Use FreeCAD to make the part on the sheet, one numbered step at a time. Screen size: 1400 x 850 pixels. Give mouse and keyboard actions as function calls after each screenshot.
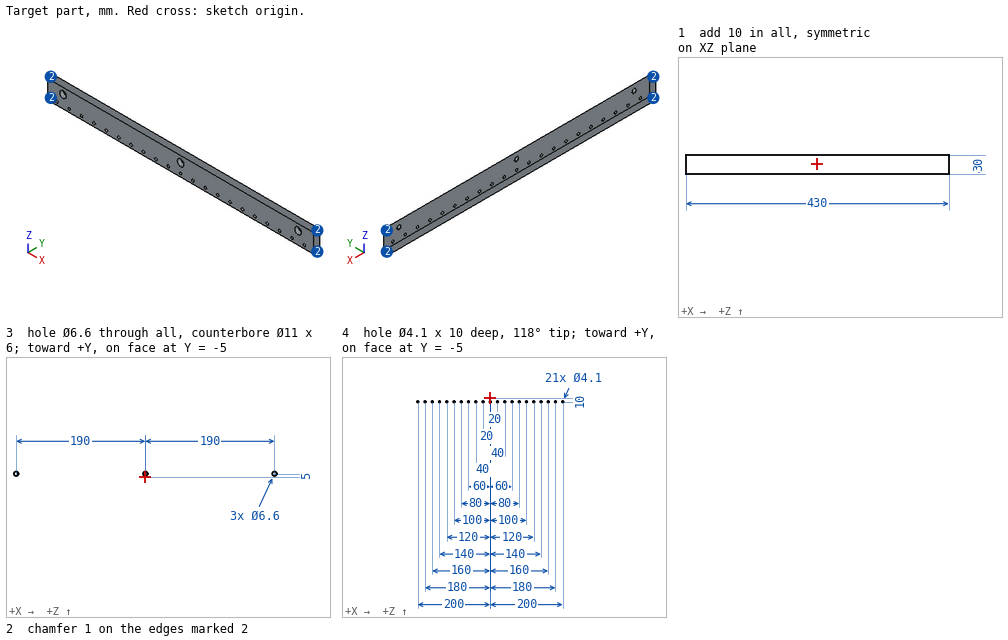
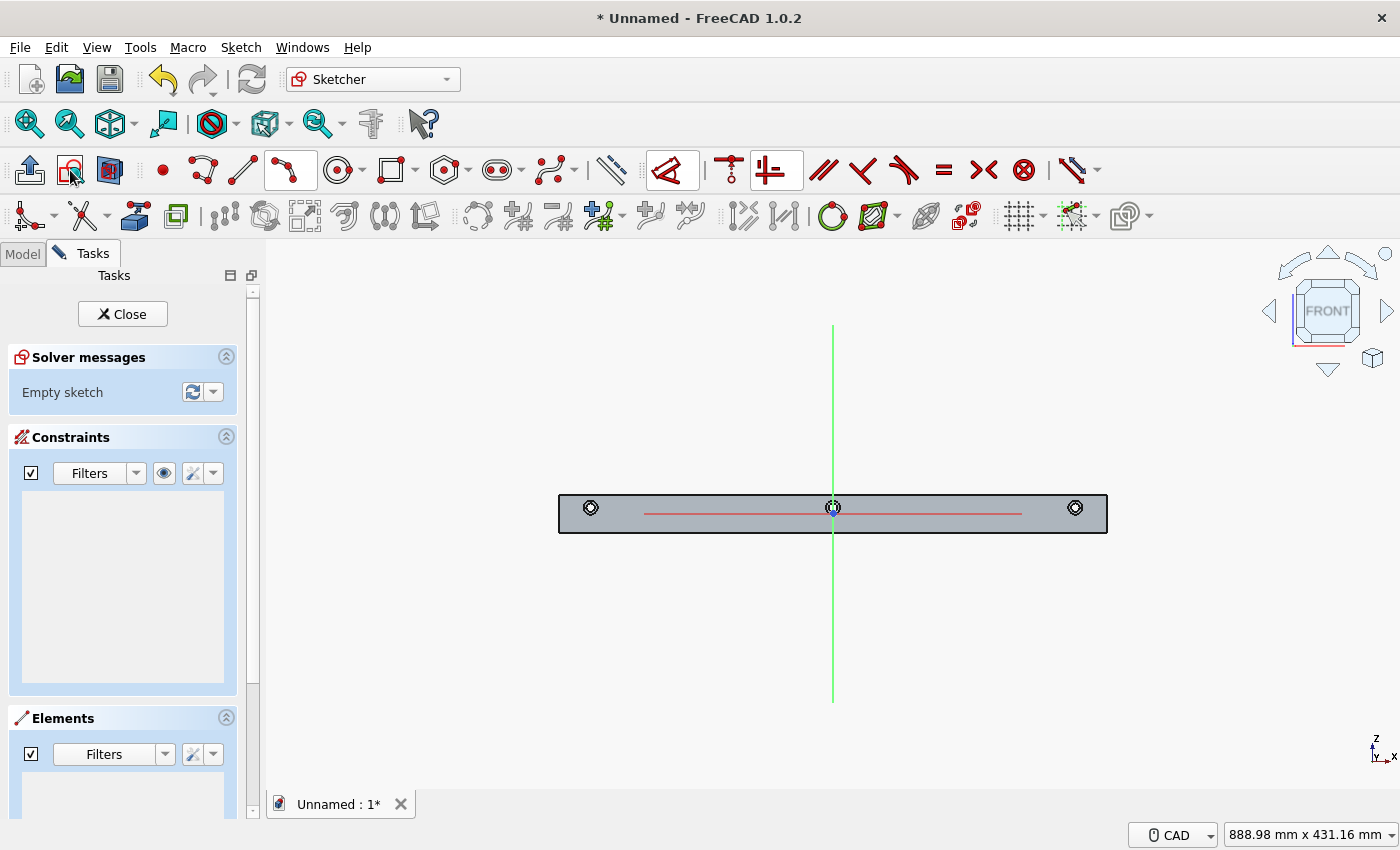
click(338, 170)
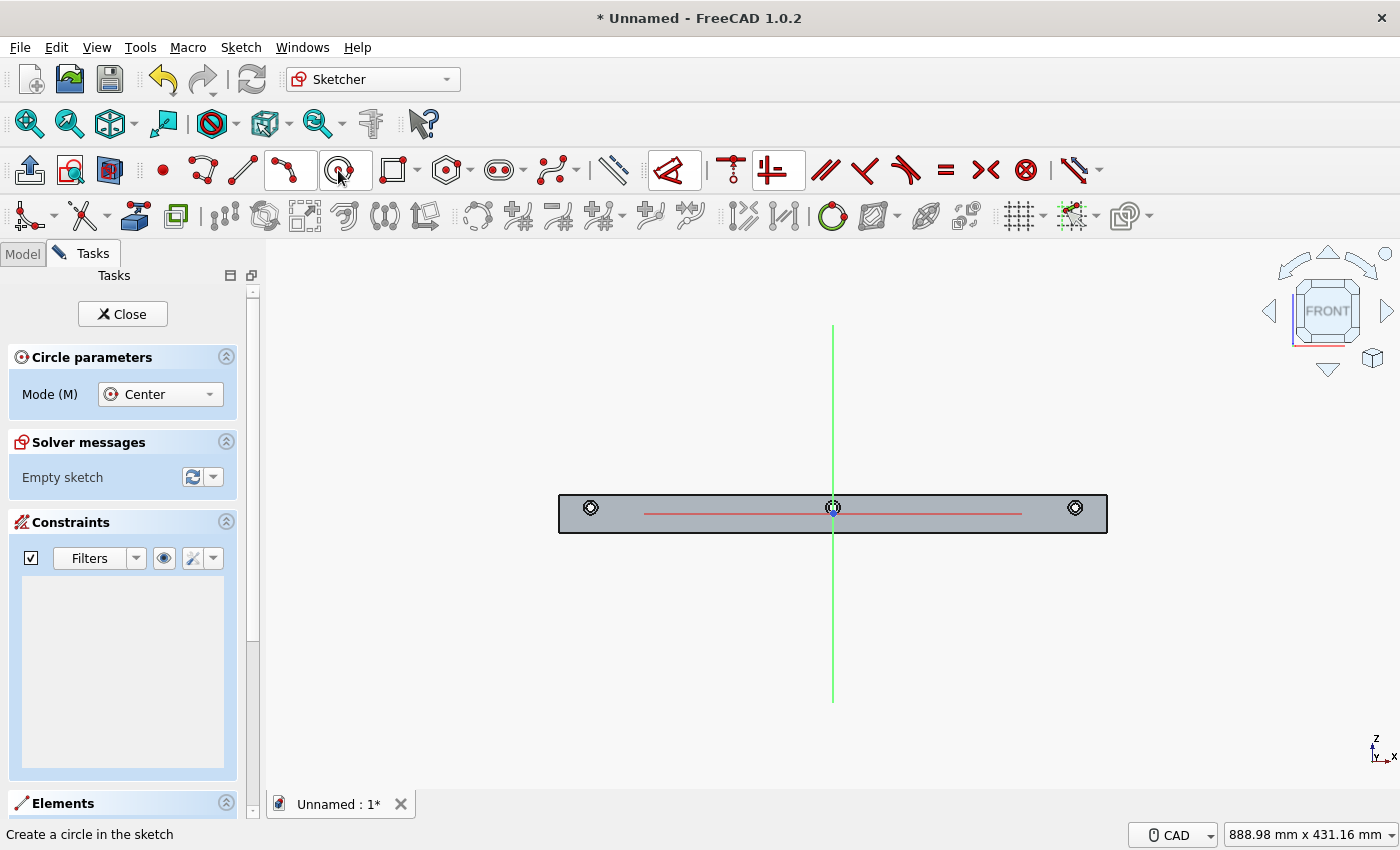
scroll(1088, 527, up, 11)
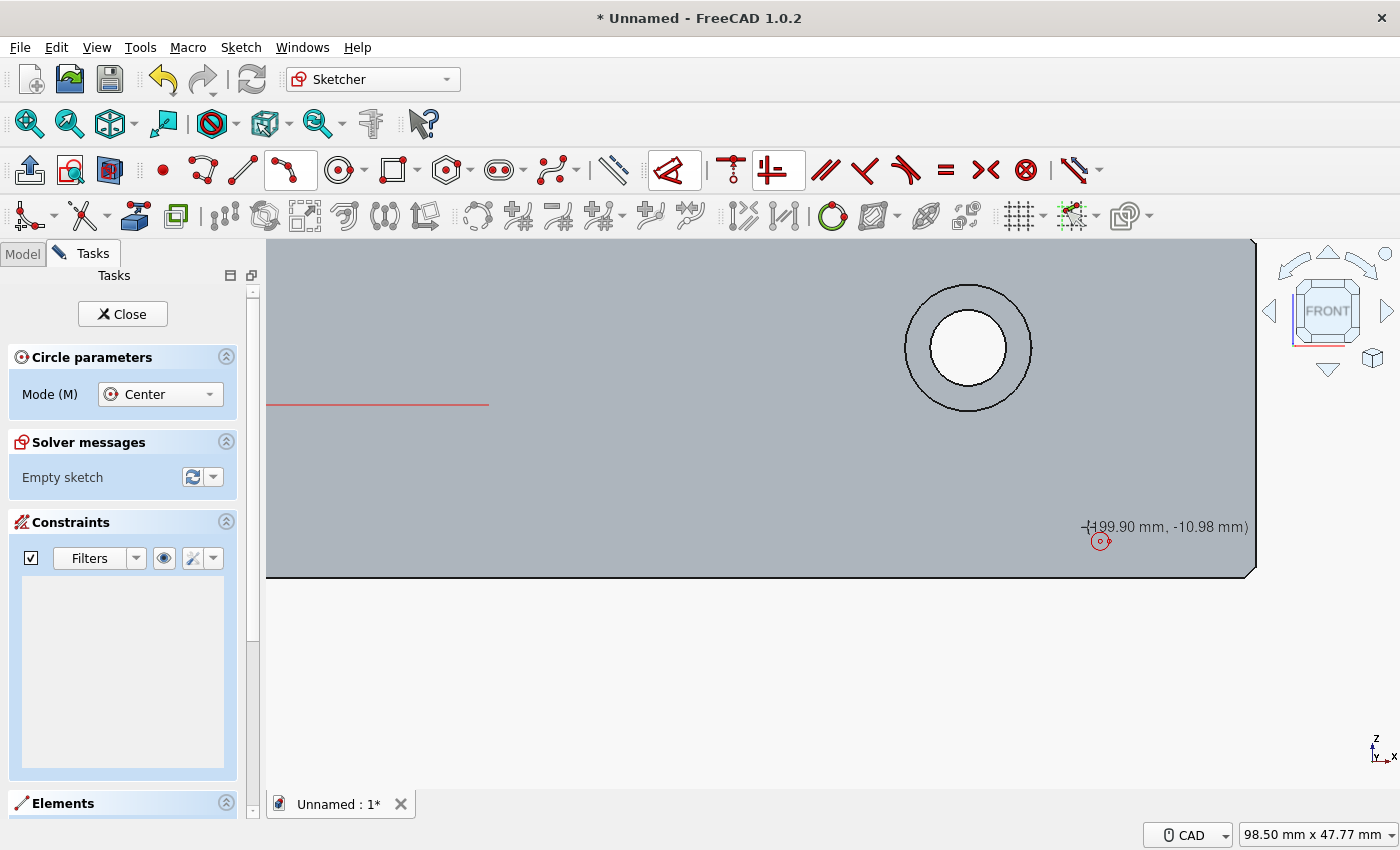
scroll(1075, 520, down, 10)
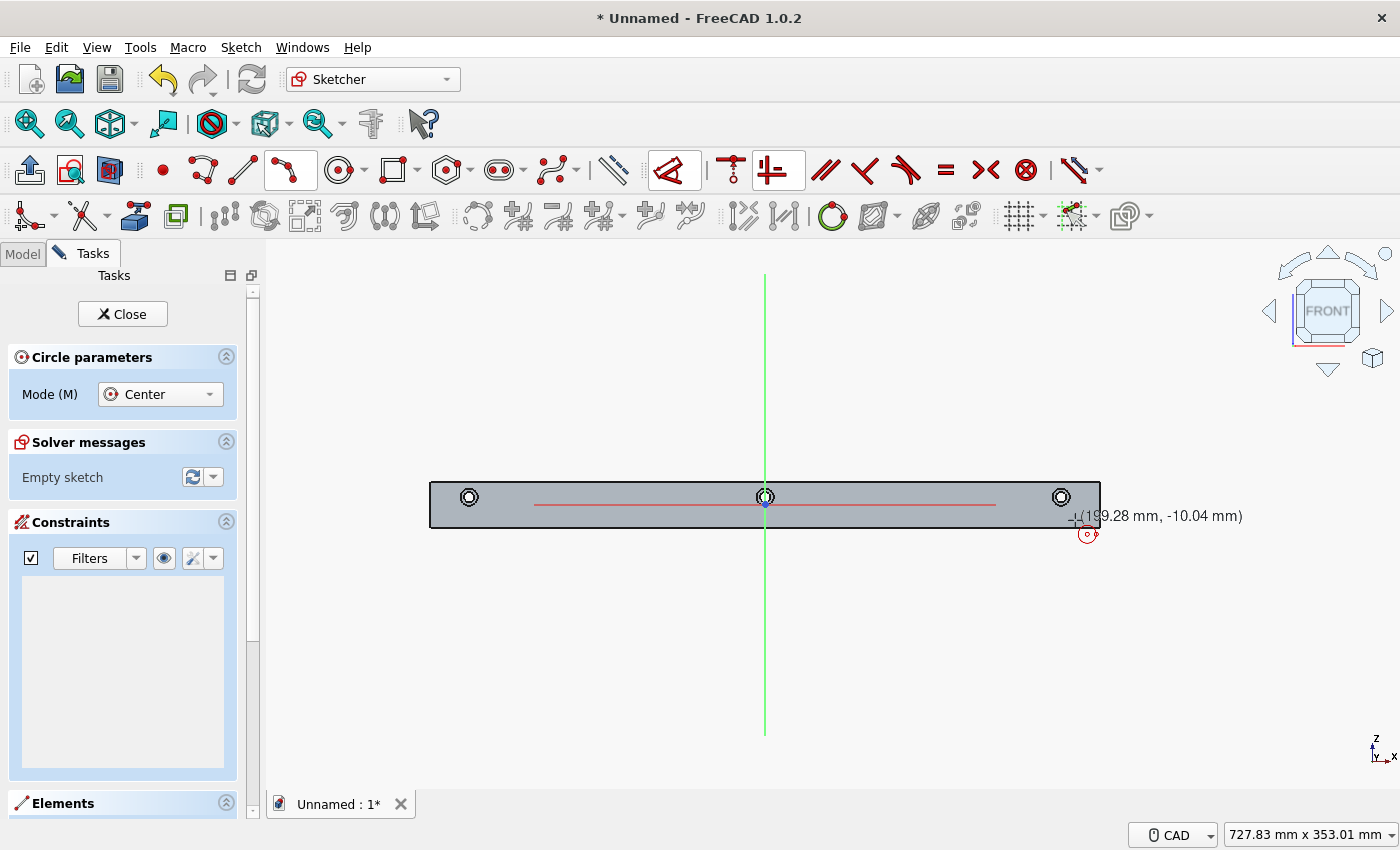
click(1077, 521)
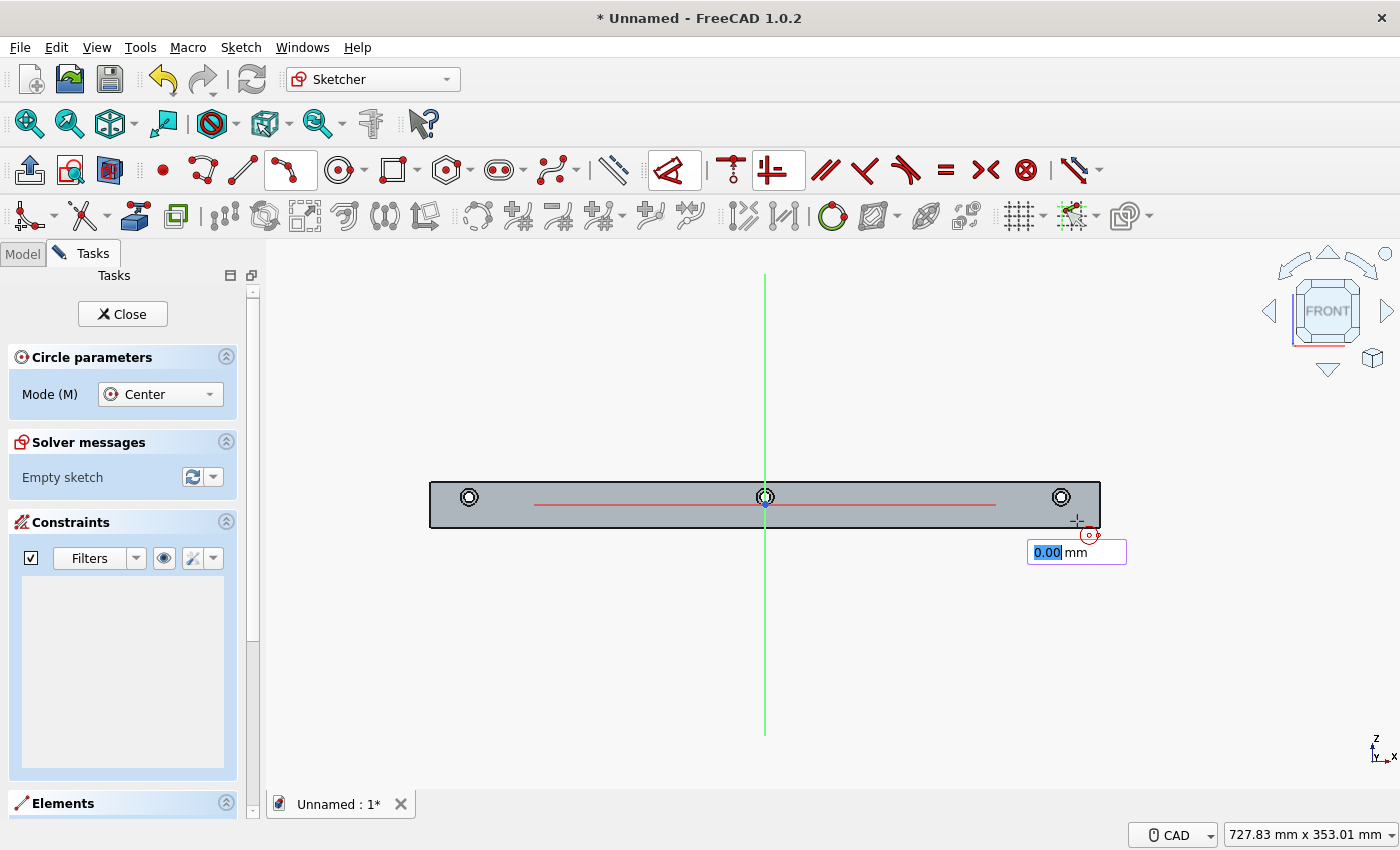
scroll(1079, 523, up, 9)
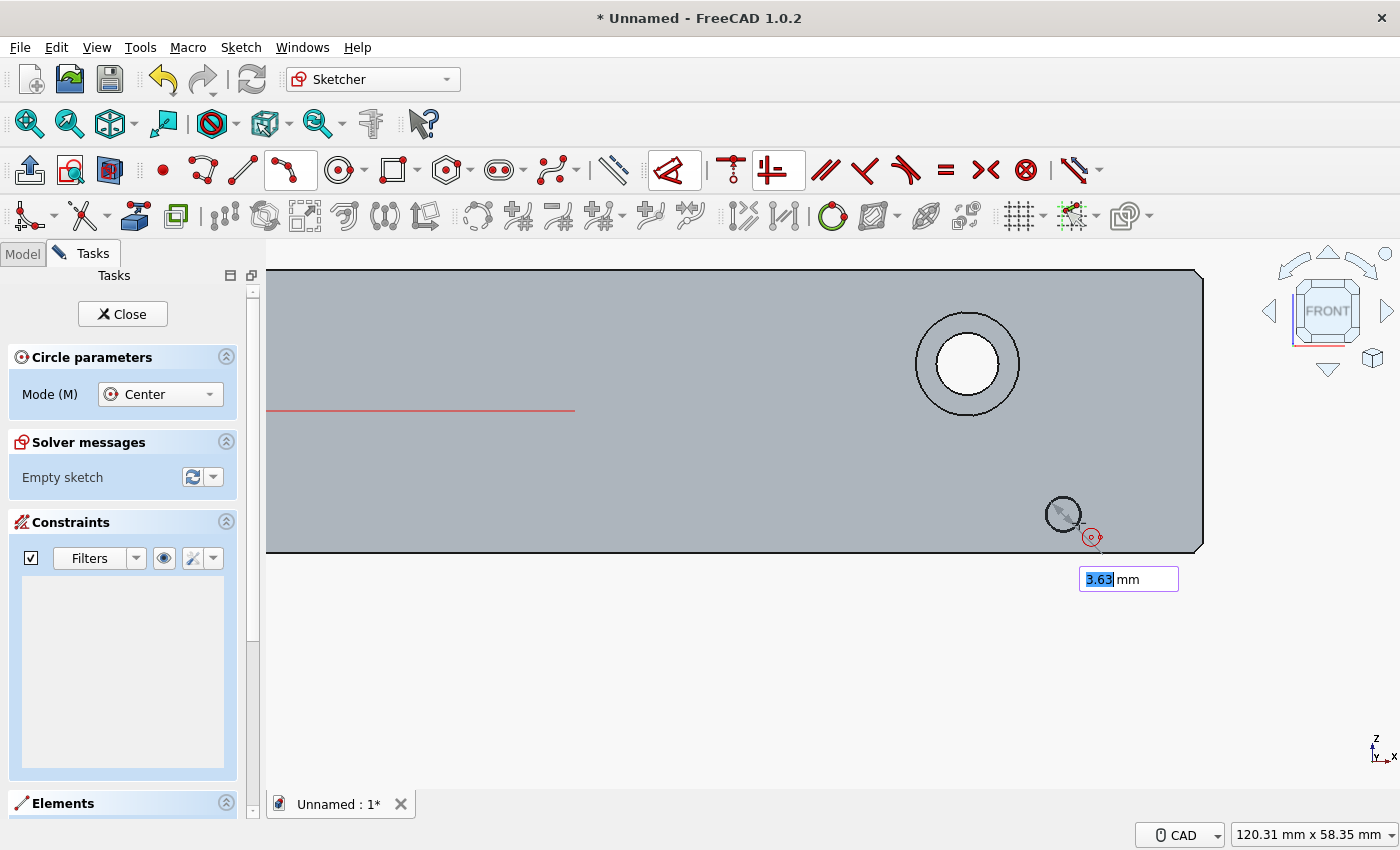
click(1075, 519)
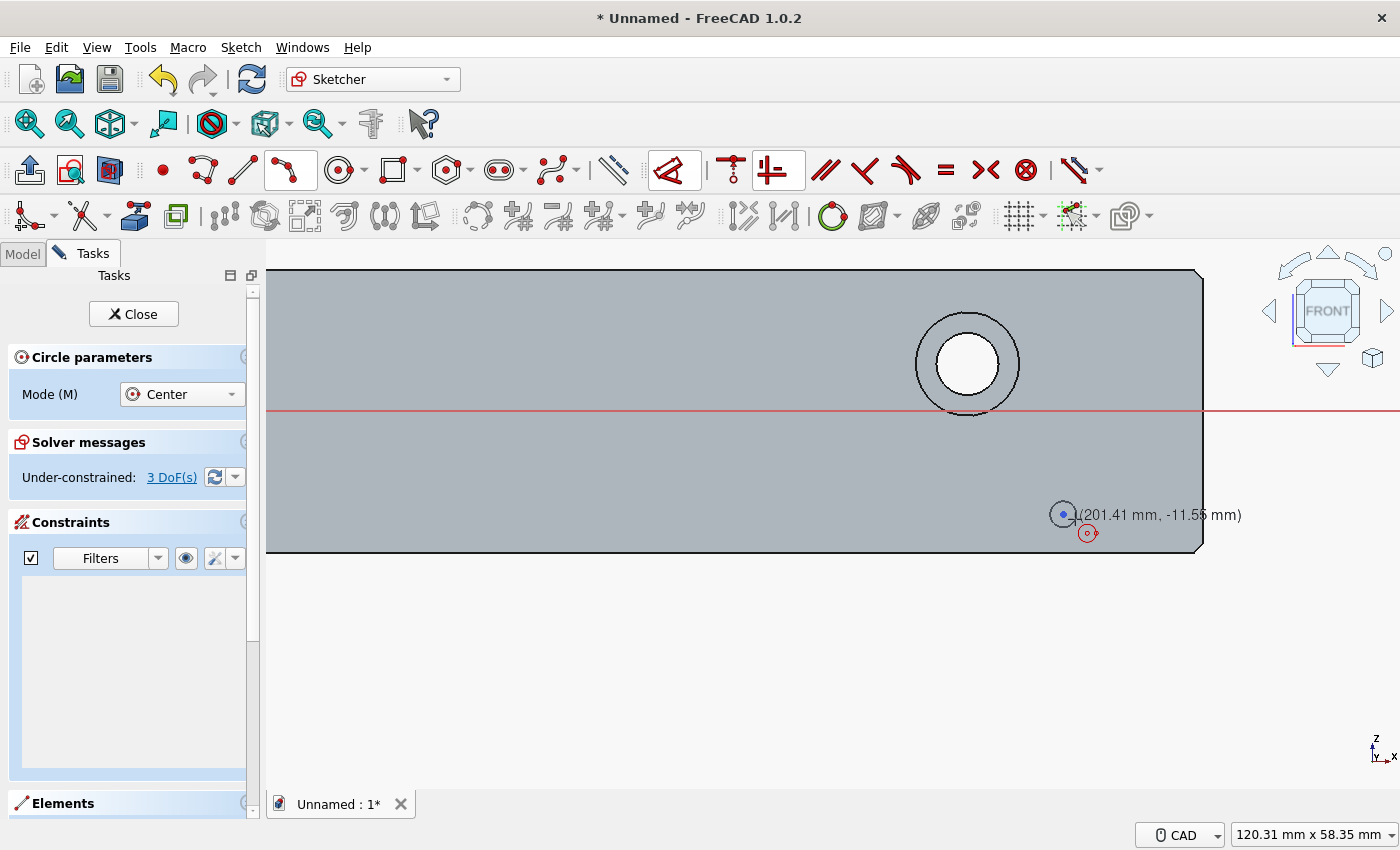
scroll(1079, 523, down, 9)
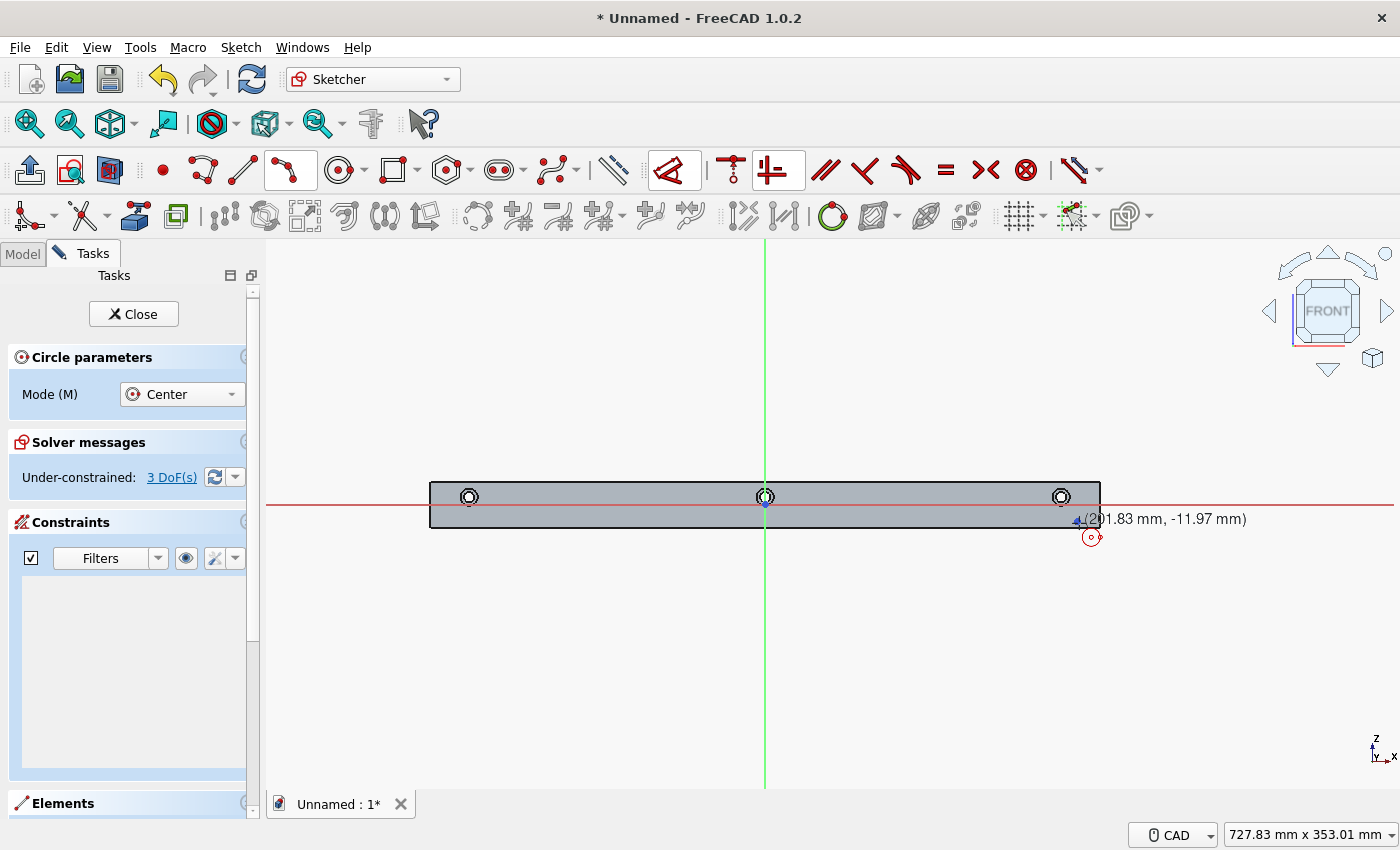
click(1046, 521)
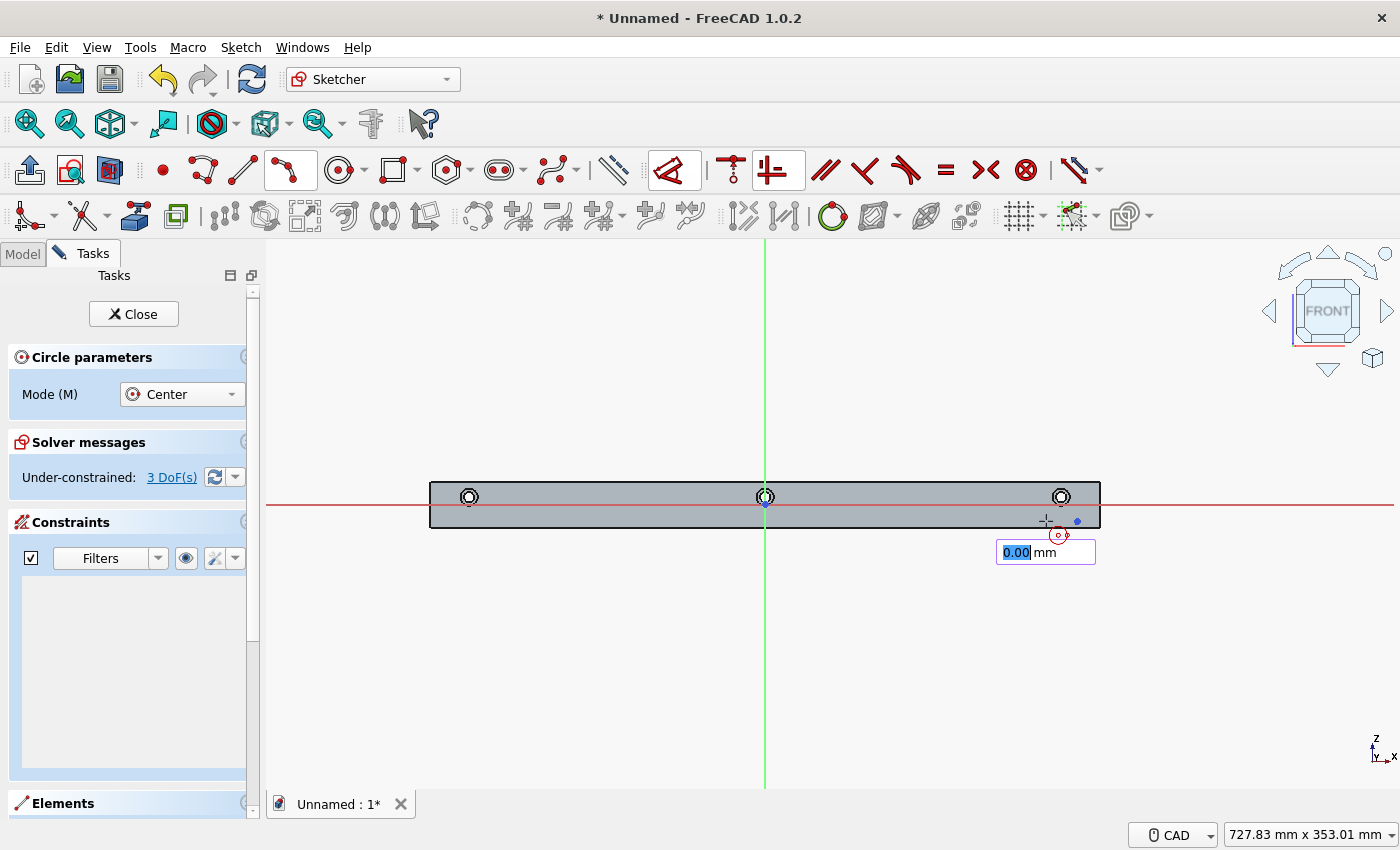
scroll(1048, 523, up, 9)